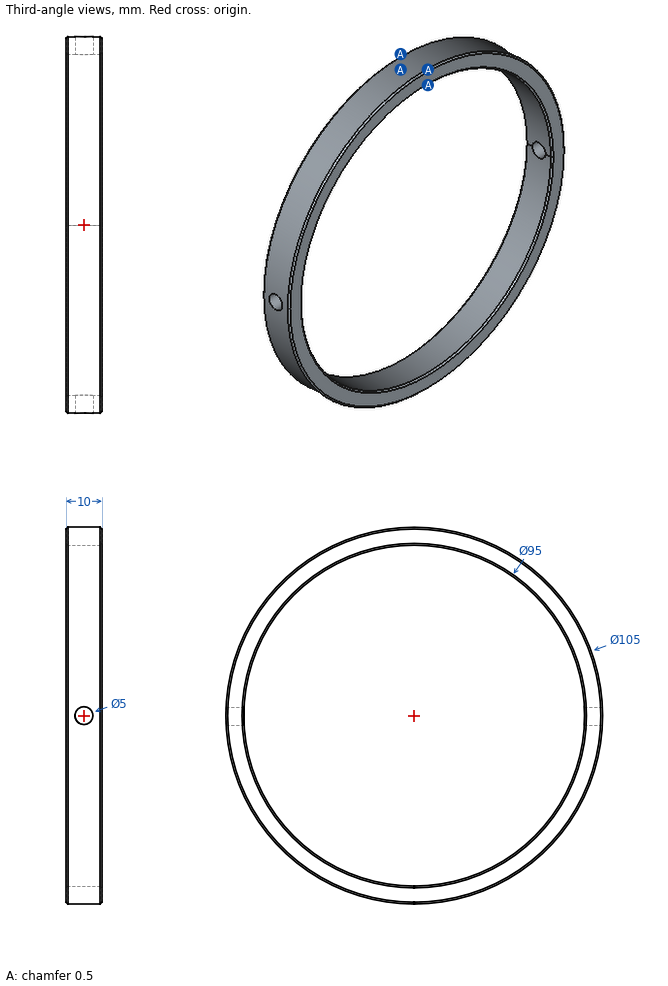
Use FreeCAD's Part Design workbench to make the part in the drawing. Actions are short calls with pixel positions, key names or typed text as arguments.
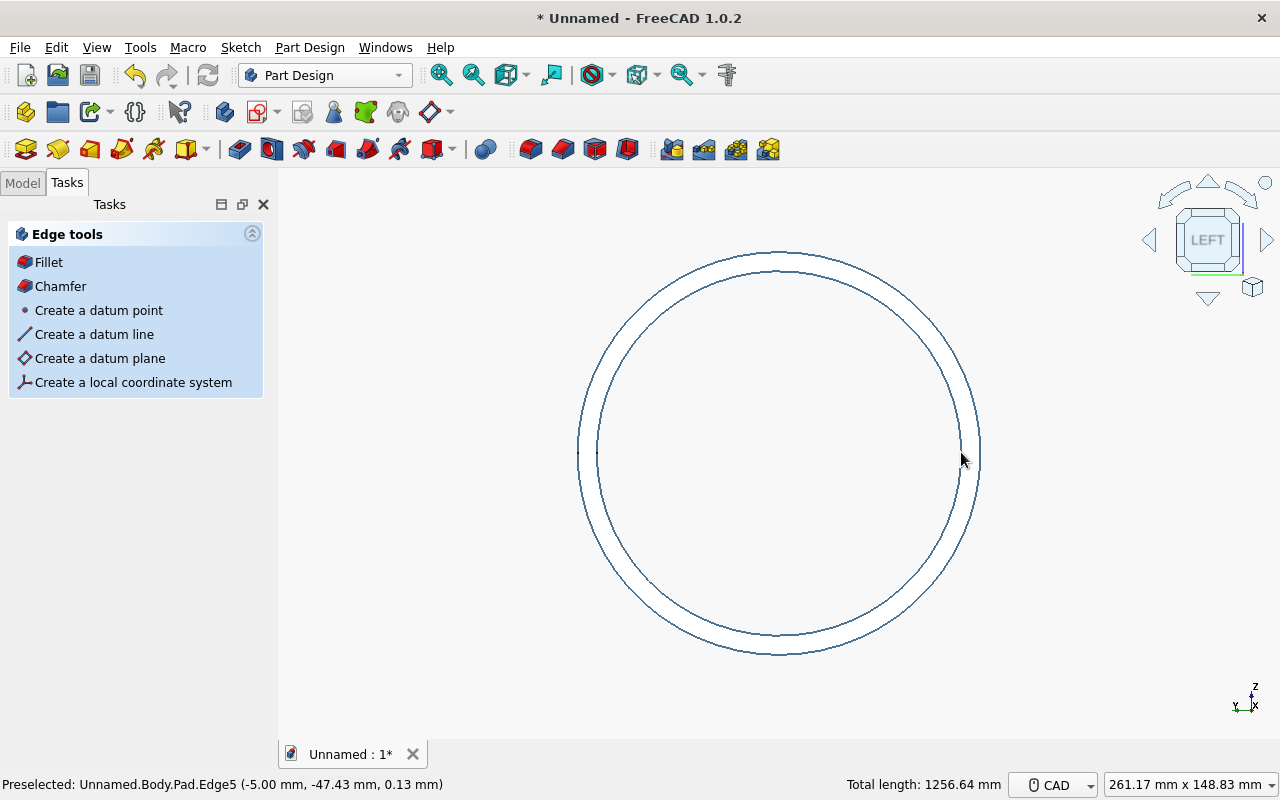
click(564, 150)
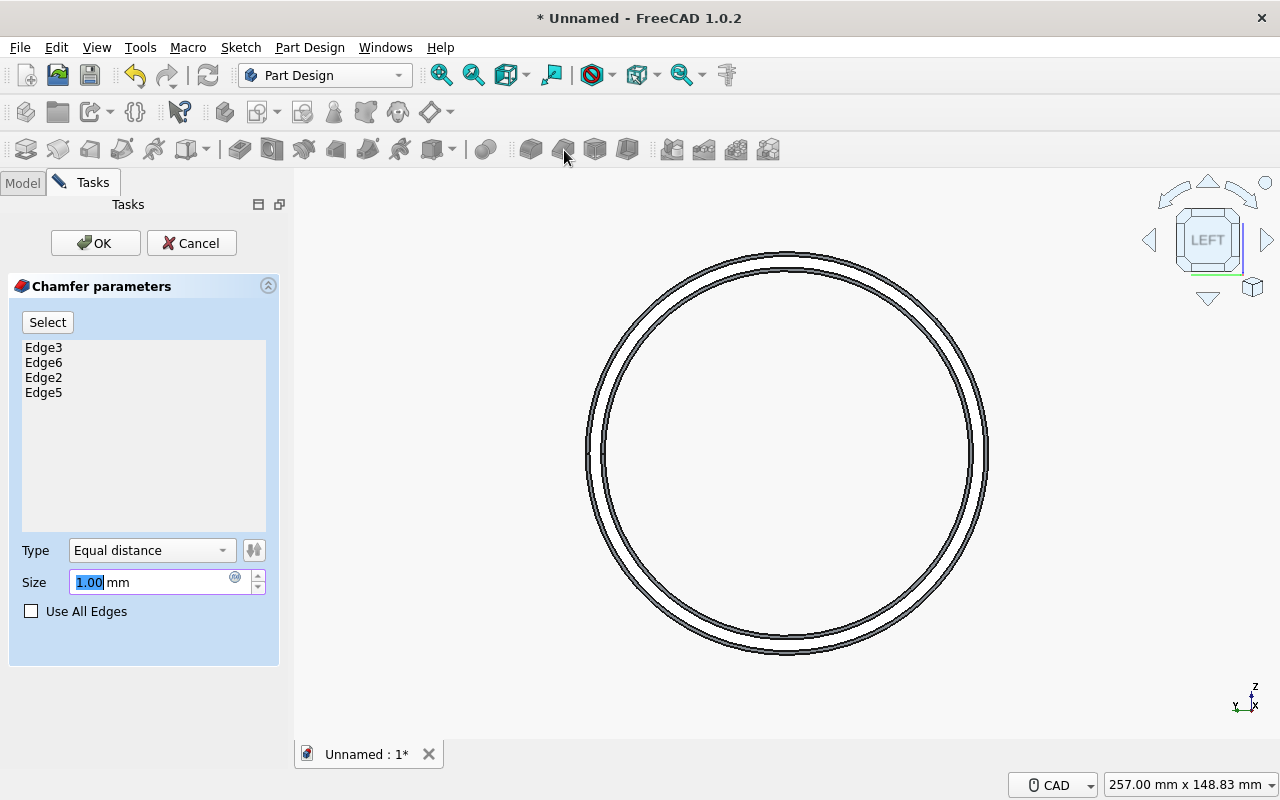
text(0.5)
key(Tab)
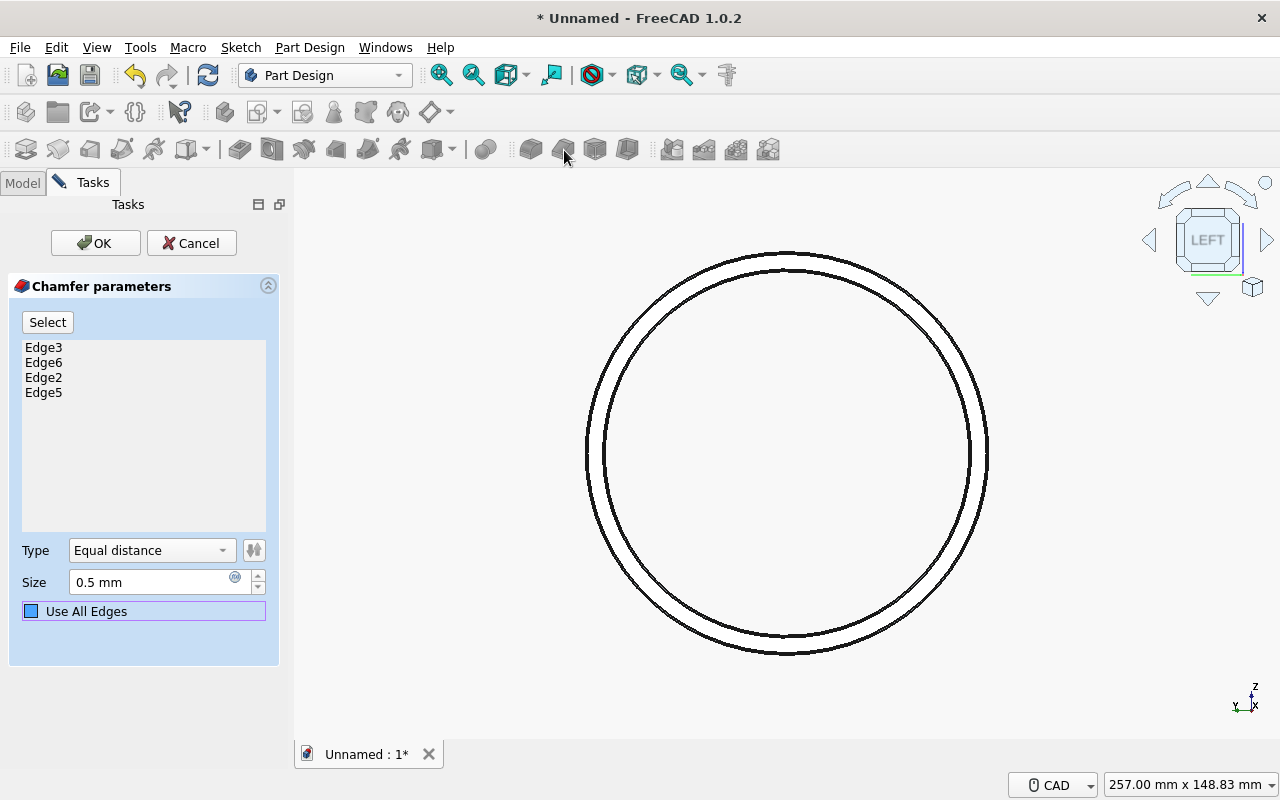
click(96, 243)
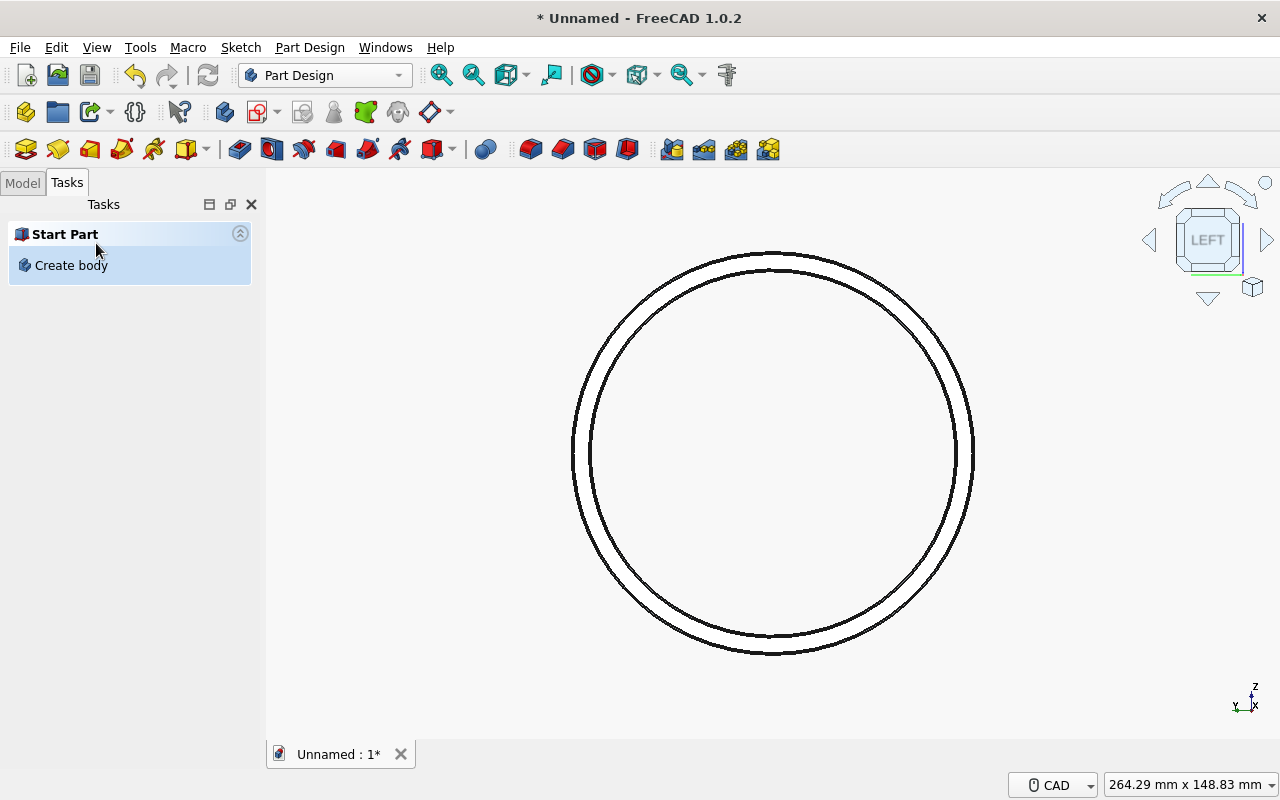
click(23, 182)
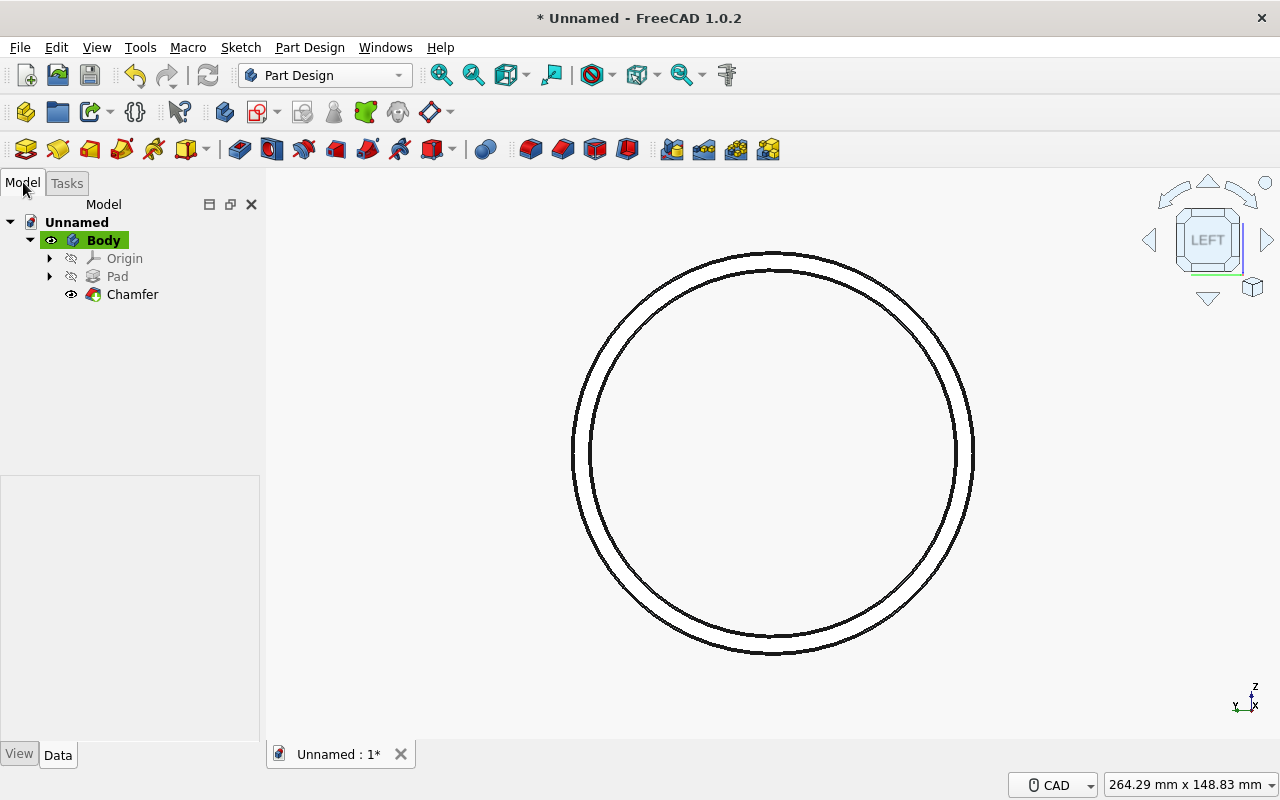
click(50, 258)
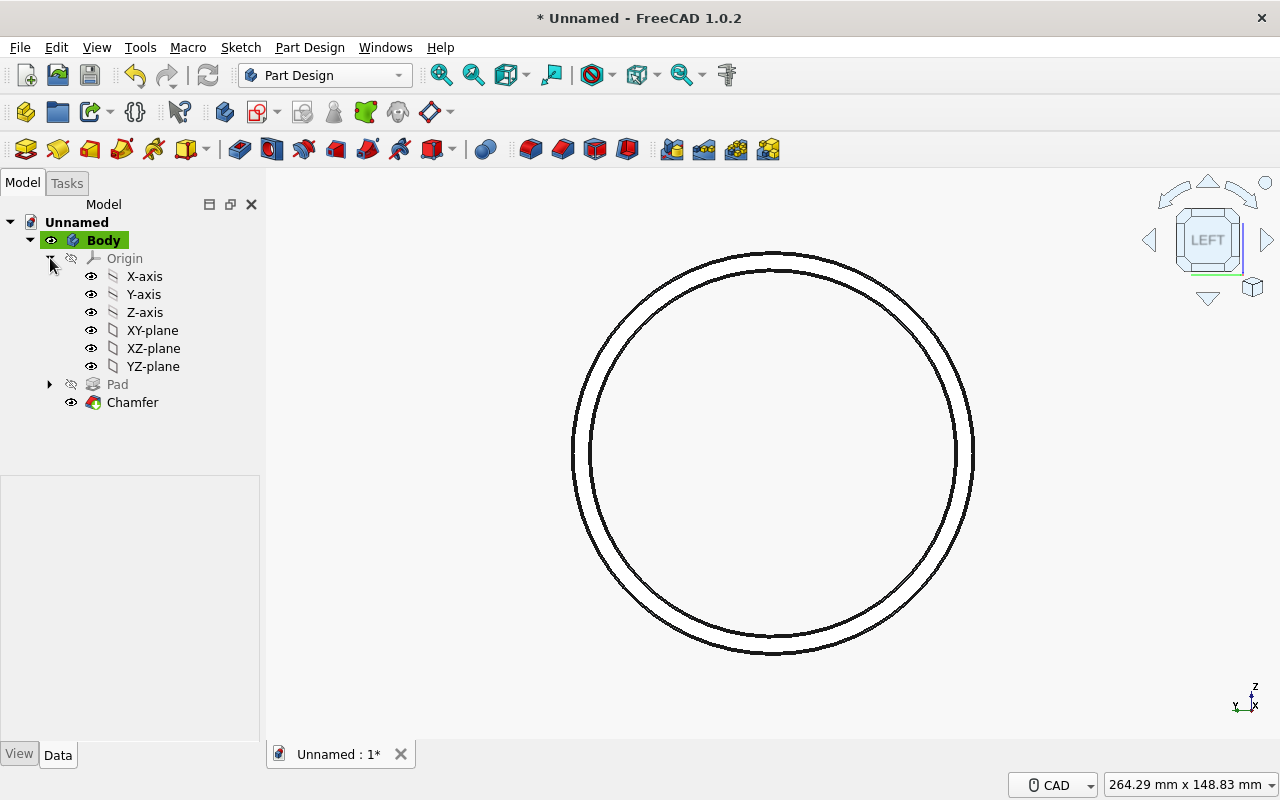
click(136, 348)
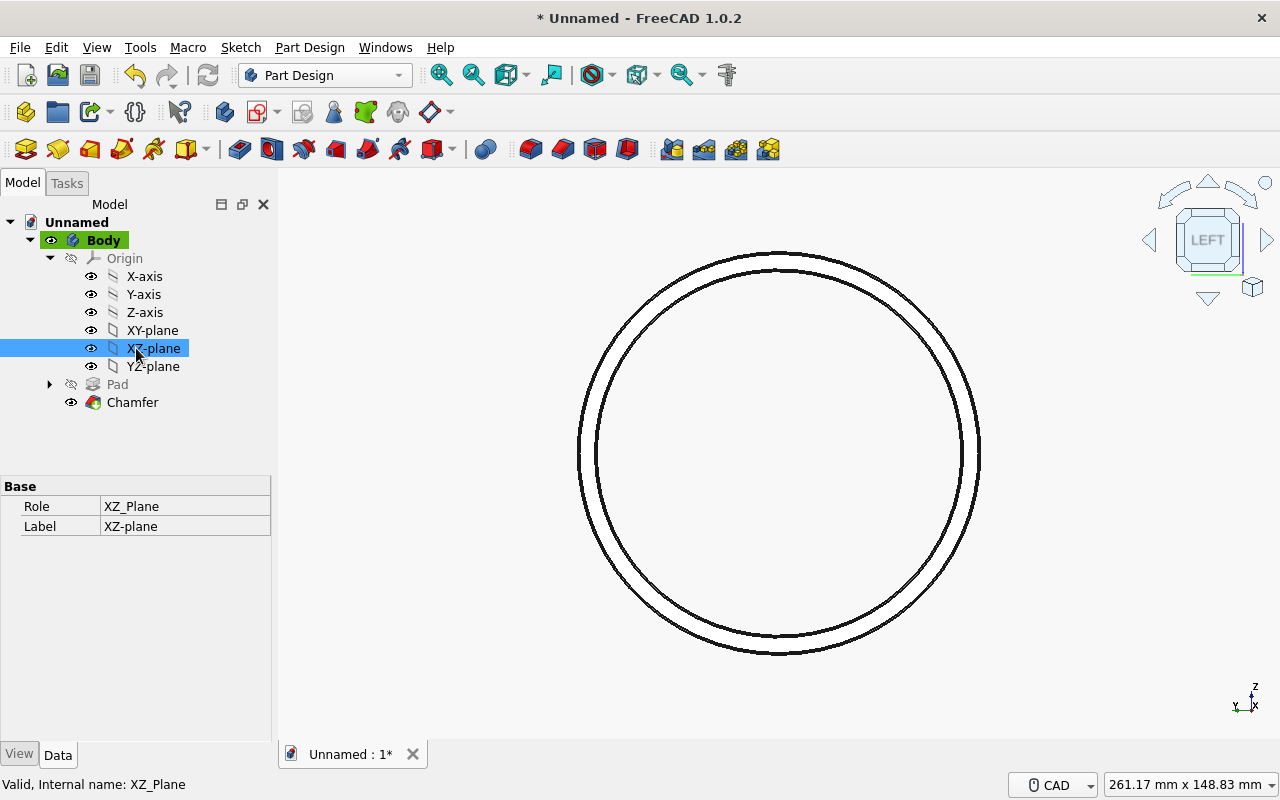
click(430, 112)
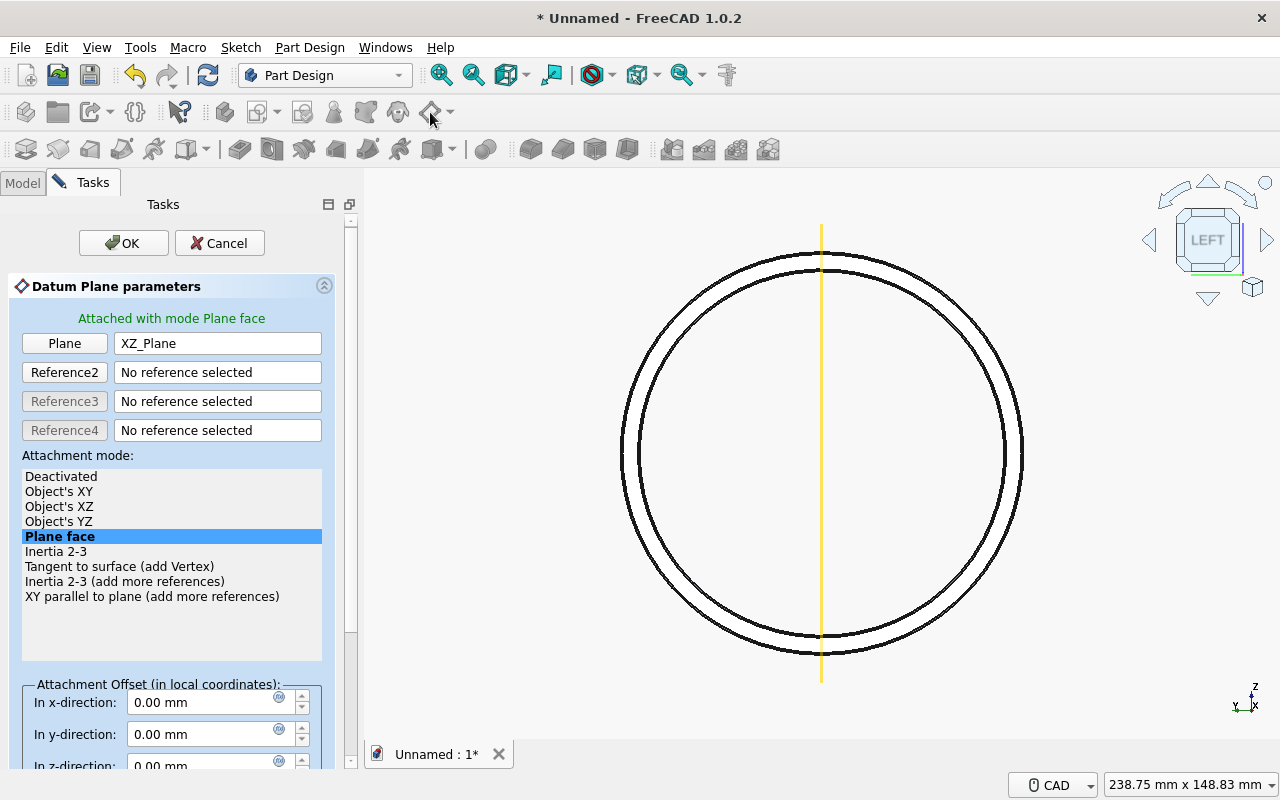
scroll(351, 491, down, 2)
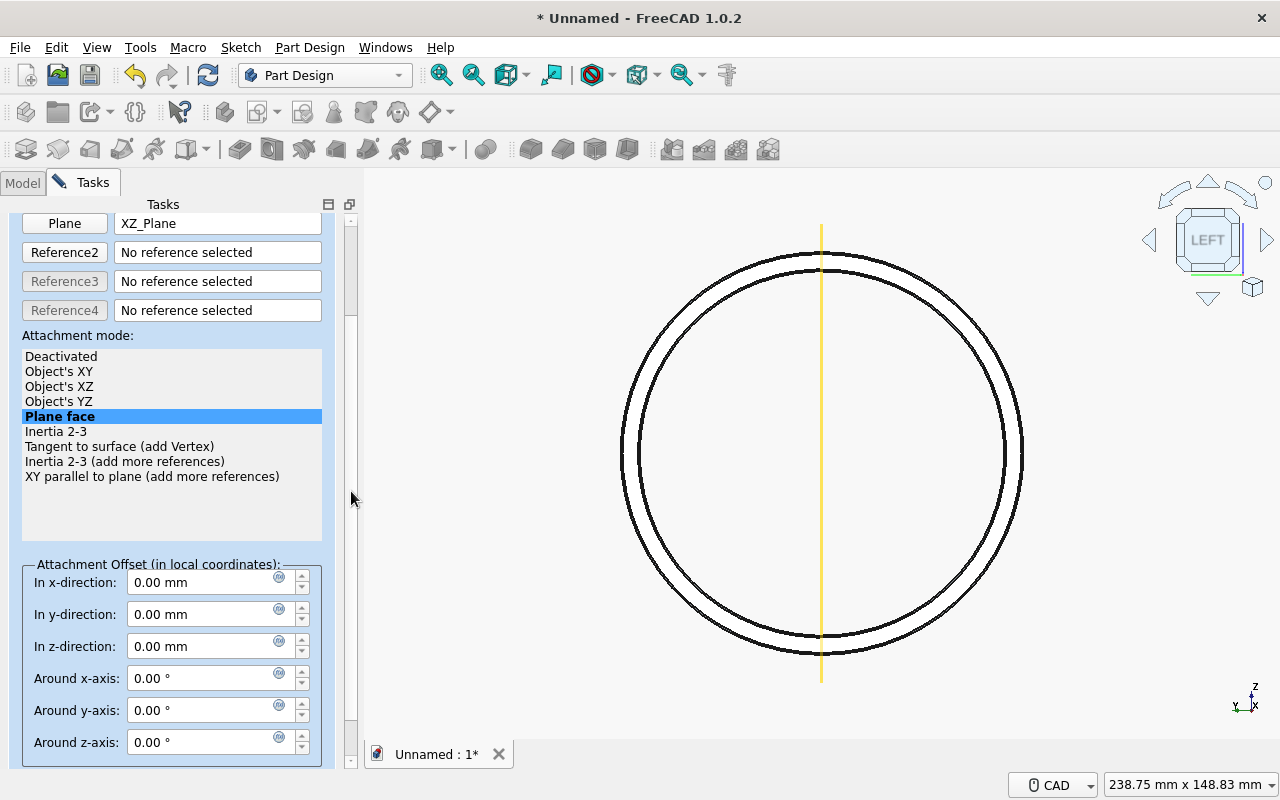
triple_click(210, 646)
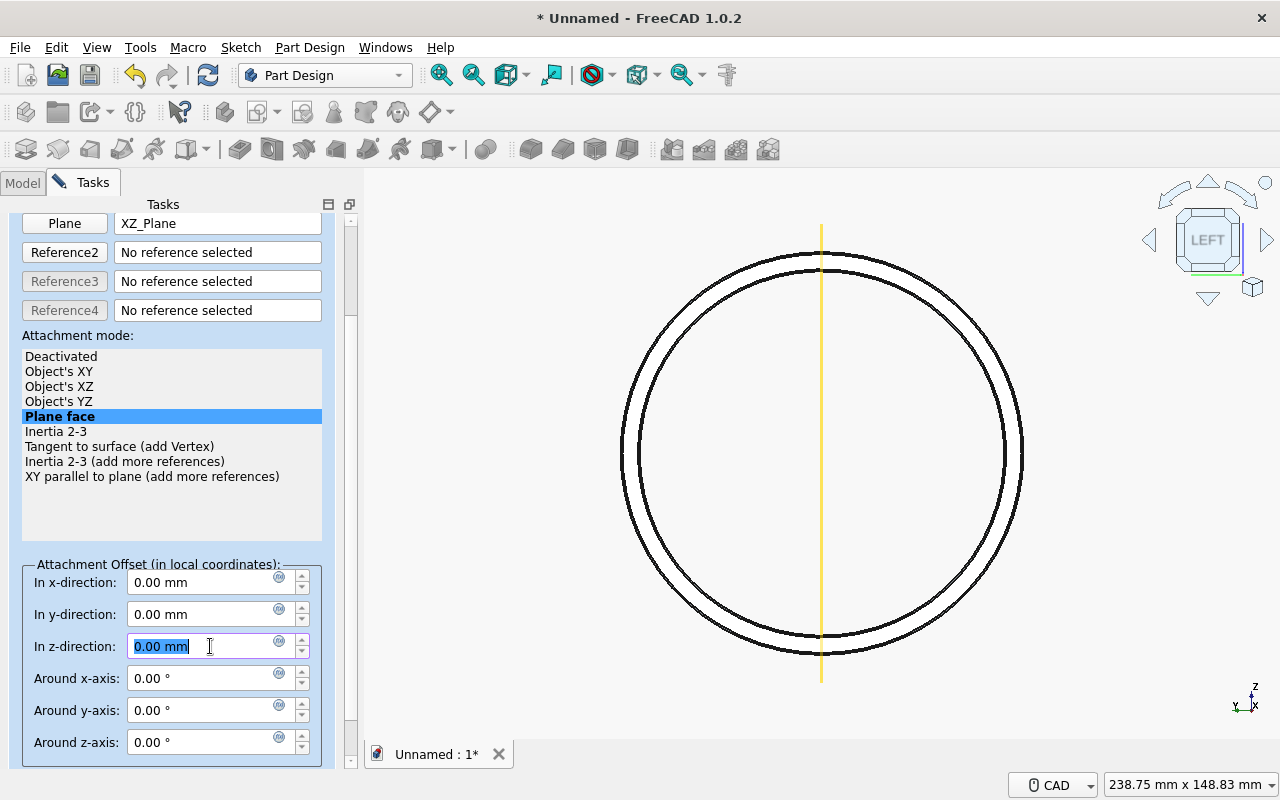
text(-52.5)
key(Tab)